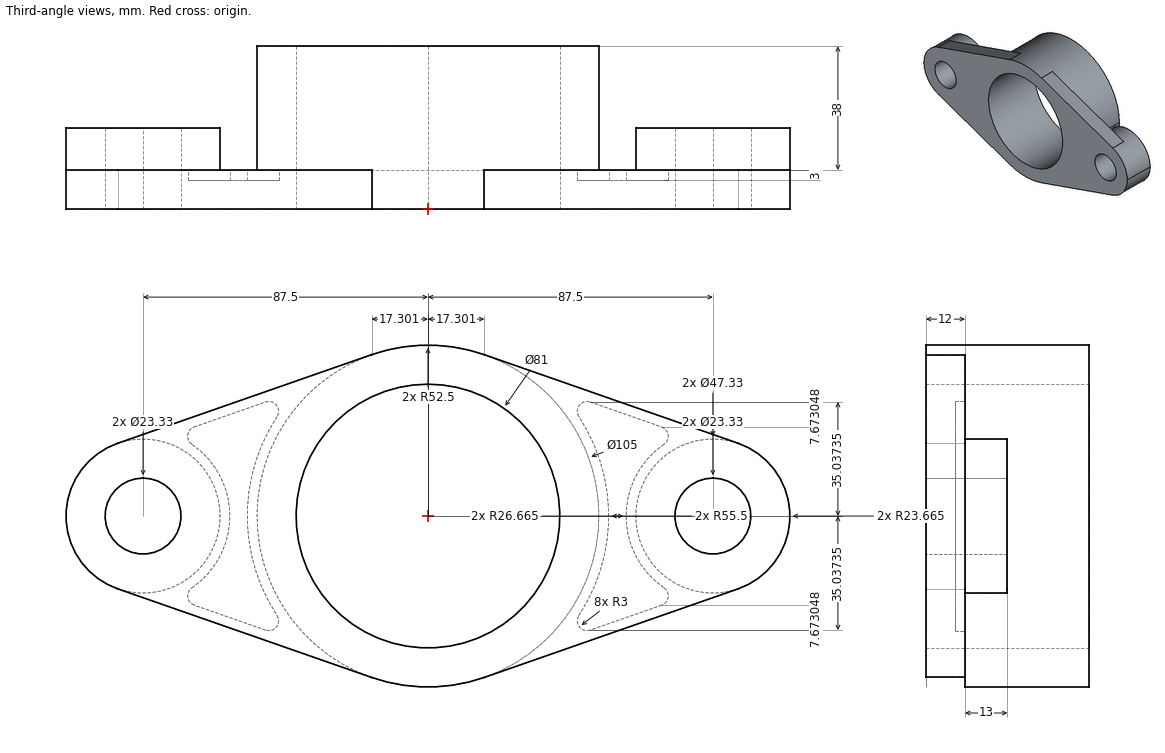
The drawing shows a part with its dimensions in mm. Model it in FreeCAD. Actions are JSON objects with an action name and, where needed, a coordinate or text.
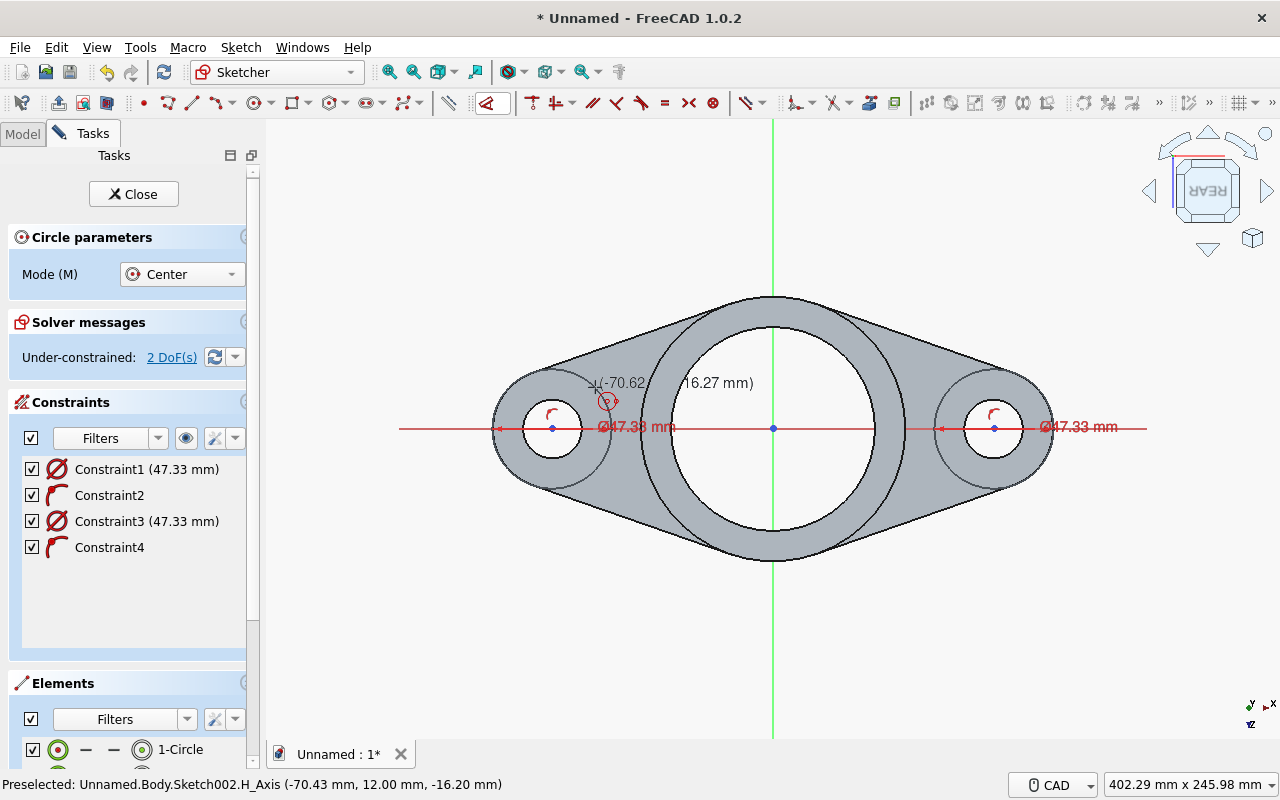
{"action": "left_click", "coordinate": [994, 429]}
{"action": "mouse_move", "coordinate": [1014, 408]}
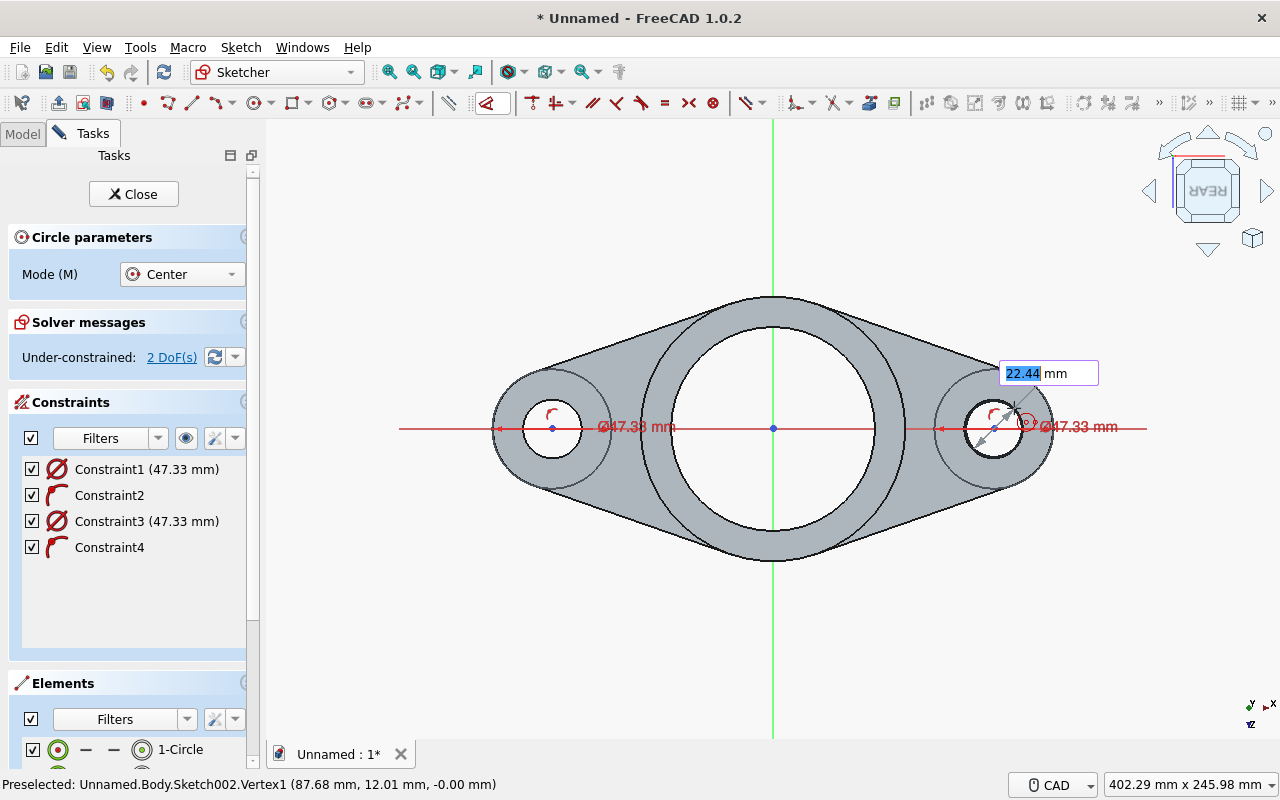
{"action": "type", "text": "23.33"}
{"action": "key", "text": "Return"}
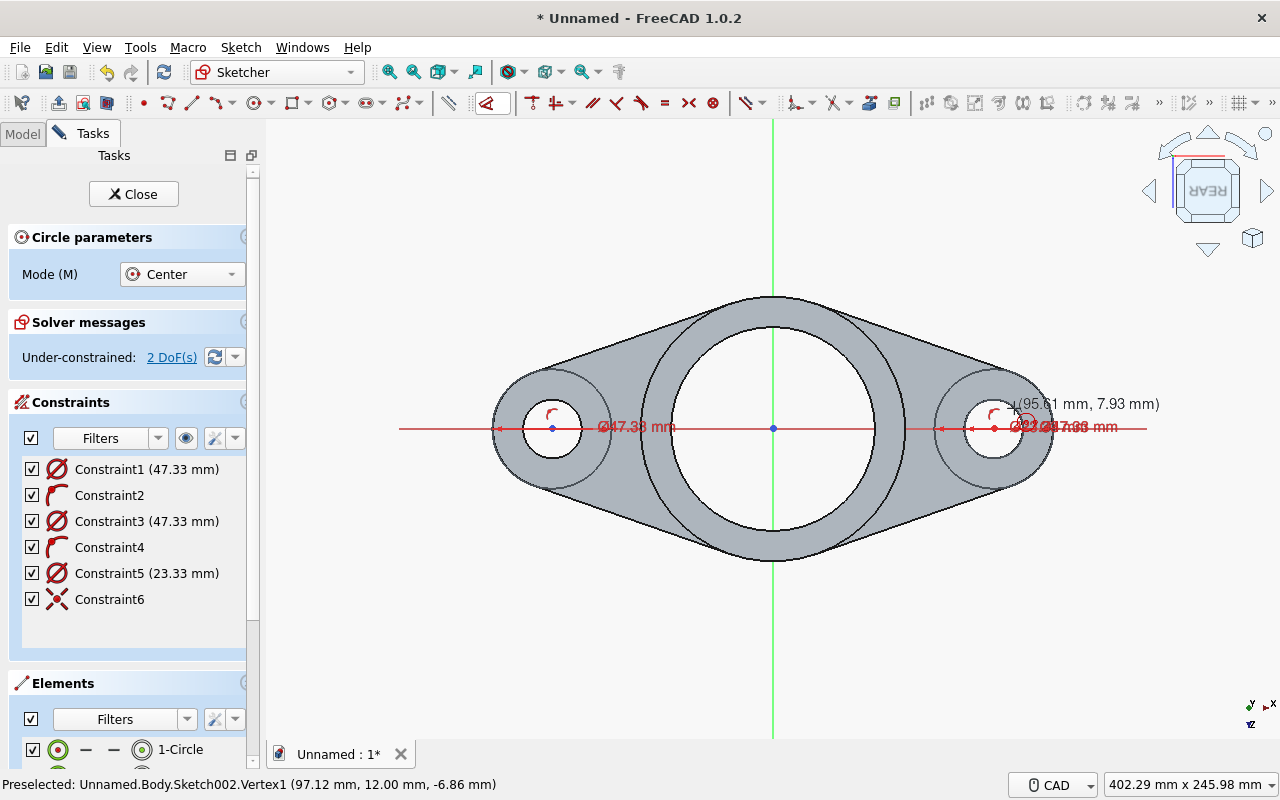
{"action": "left_click", "coordinate": [552, 429]}
{"action": "mouse_move", "coordinate": [573, 408]}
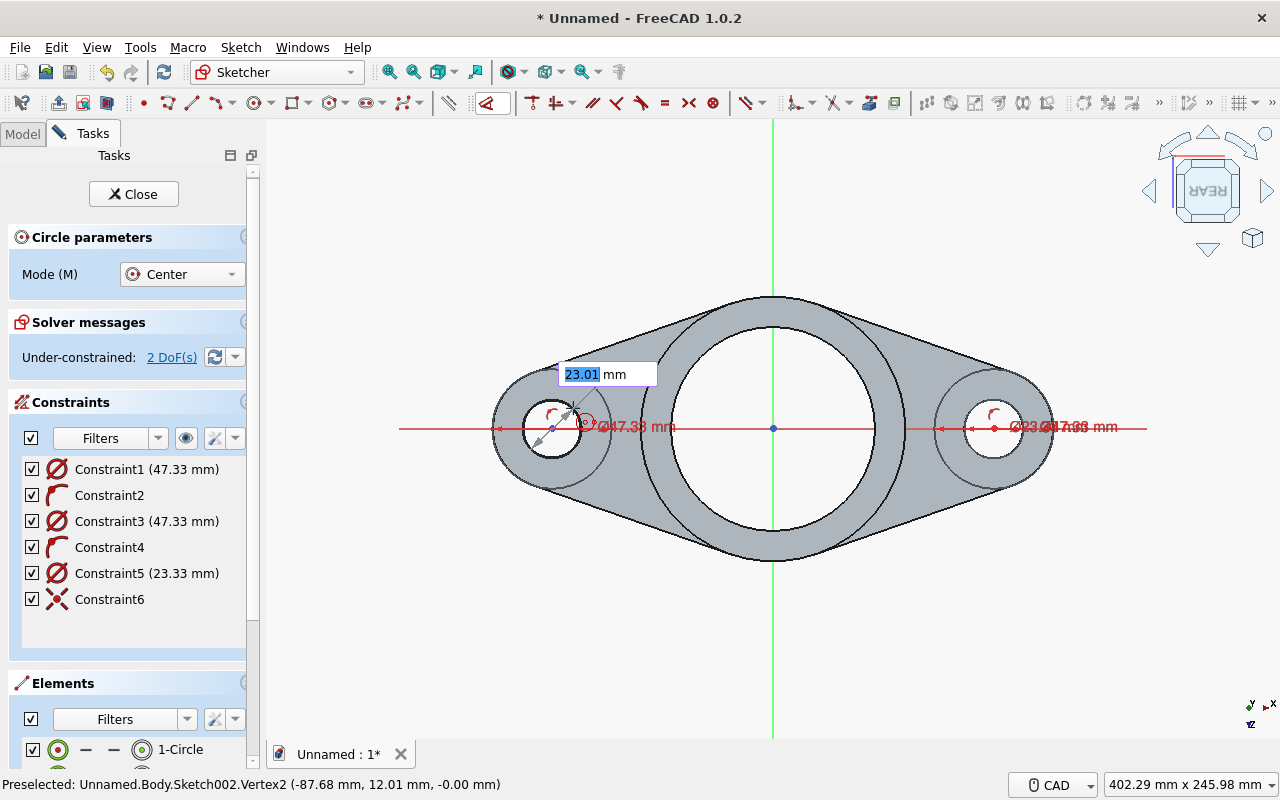
{"action": "type", "text": "23.33"}
{"action": "key", "text": "Return"}
{"action": "key", "text": "Escape"}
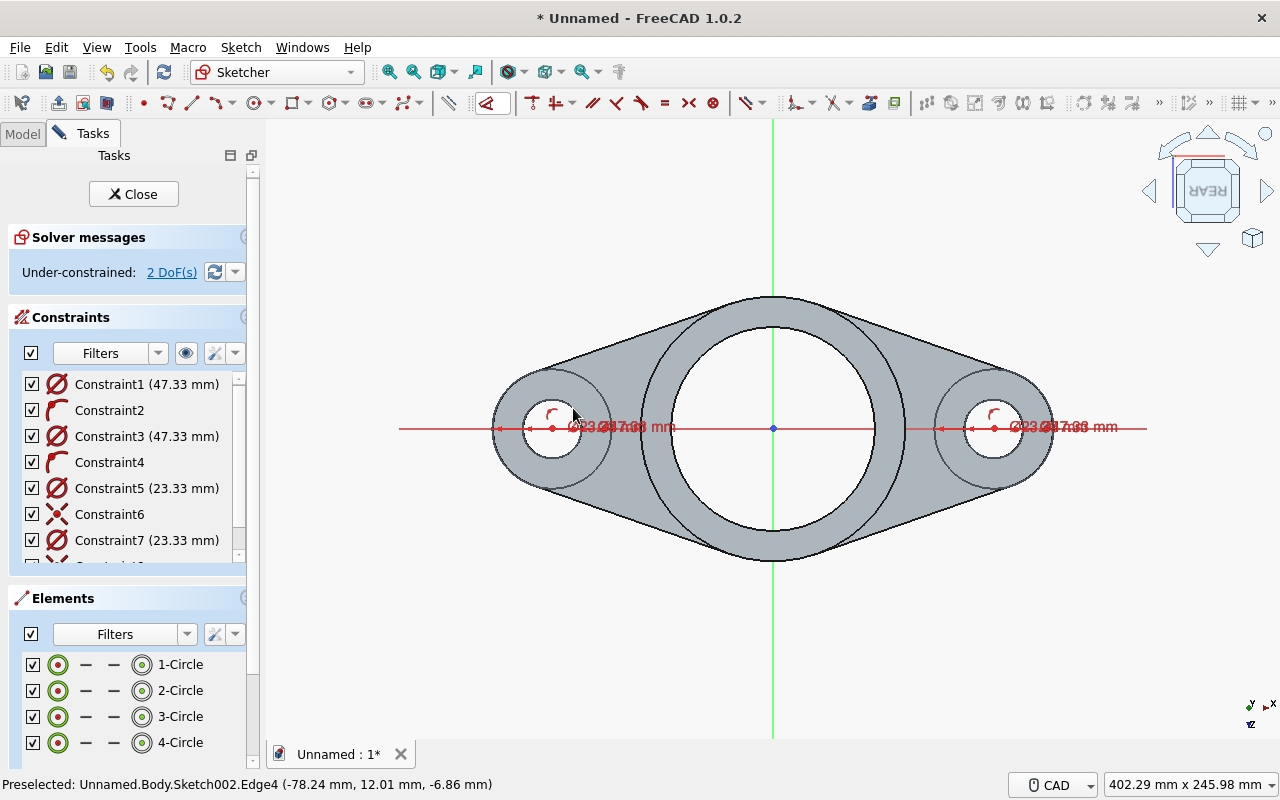
{"action": "left_click", "coordinate": [994, 429]}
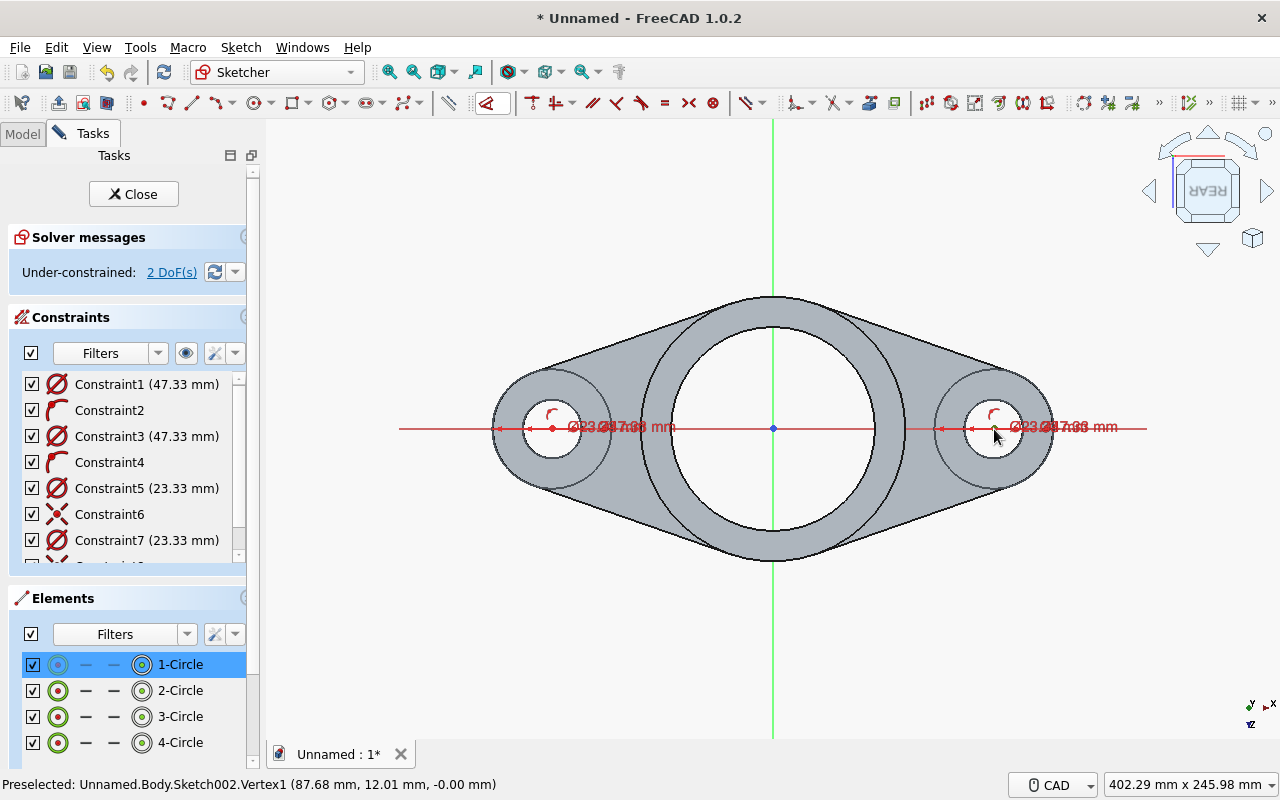
{"action": "left_click", "coordinate": [504, 104]}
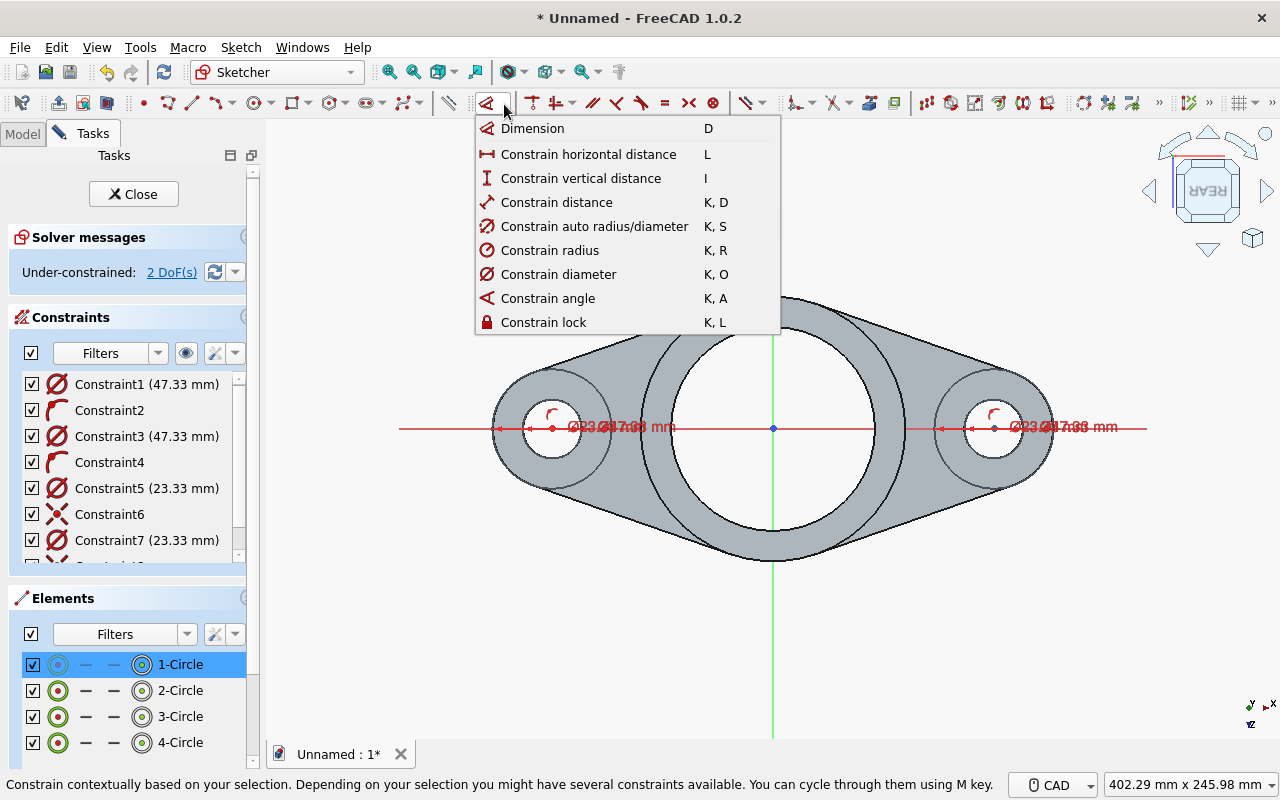
{"action": "left_click", "coordinate": [628, 154]}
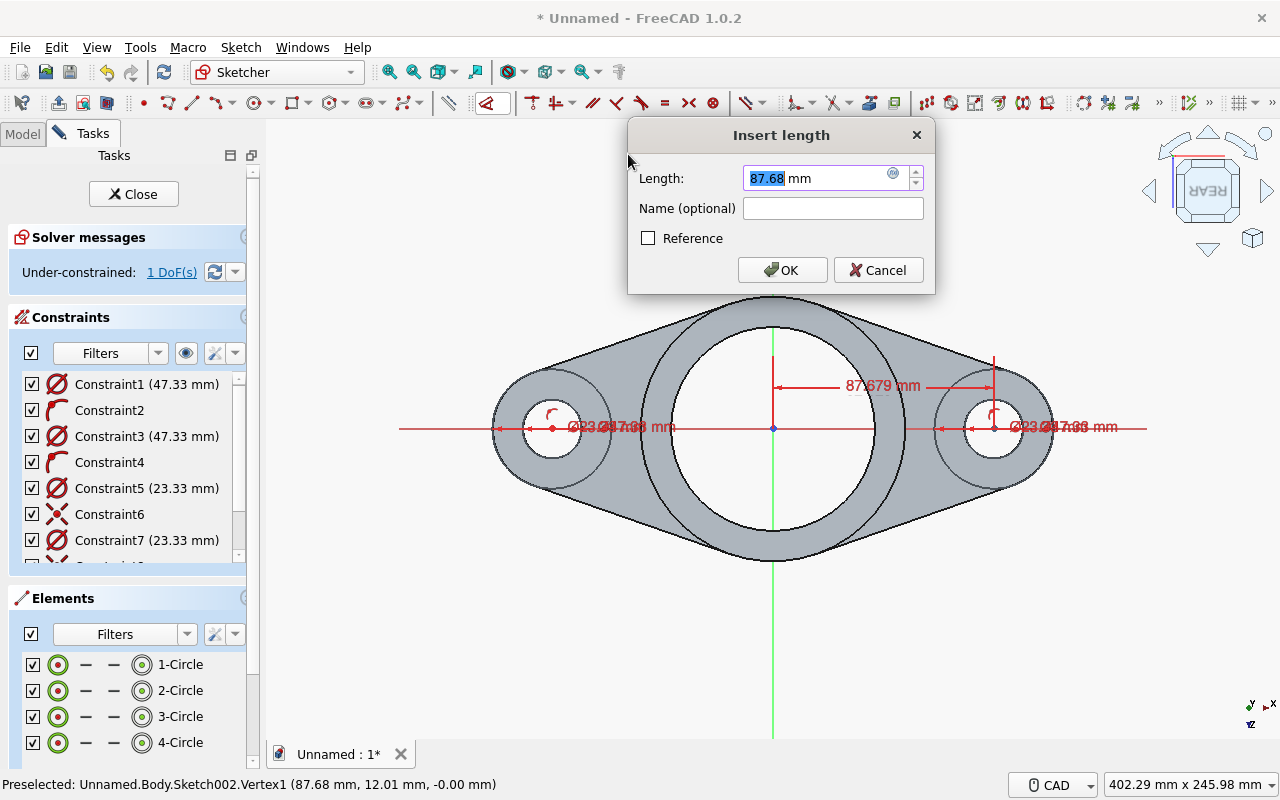
{"action": "type", "text": "87.5"}
{"action": "key", "text": "Return"}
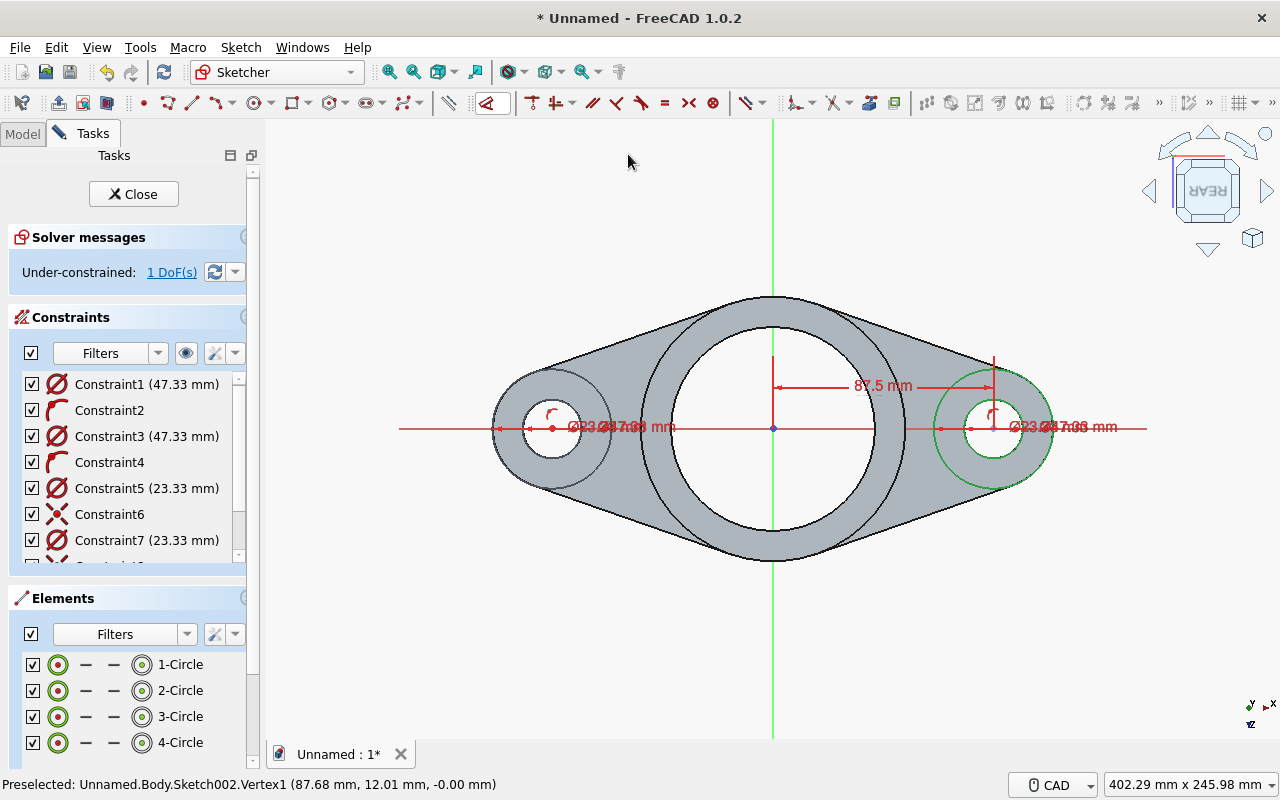
{"action": "left_click", "coordinate": [552, 429]}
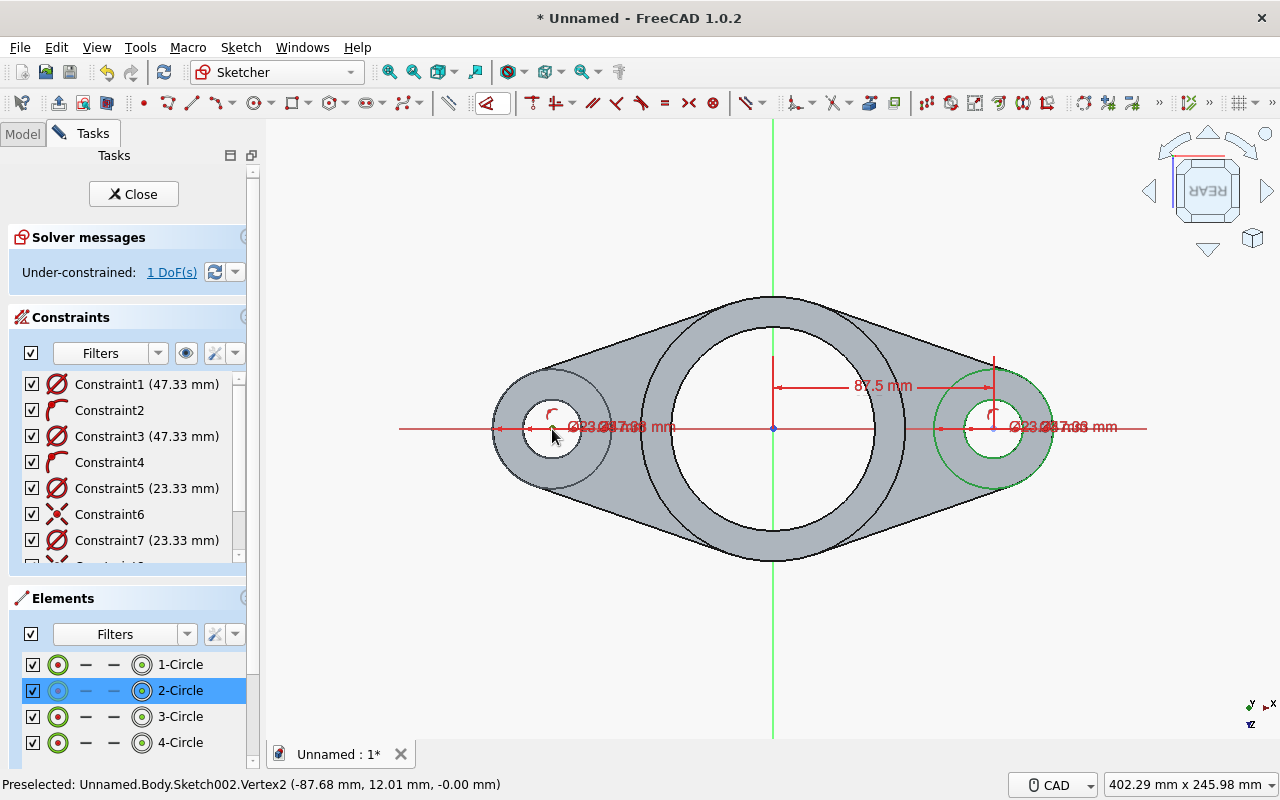
{"action": "left_click", "coordinate": [504, 104]}